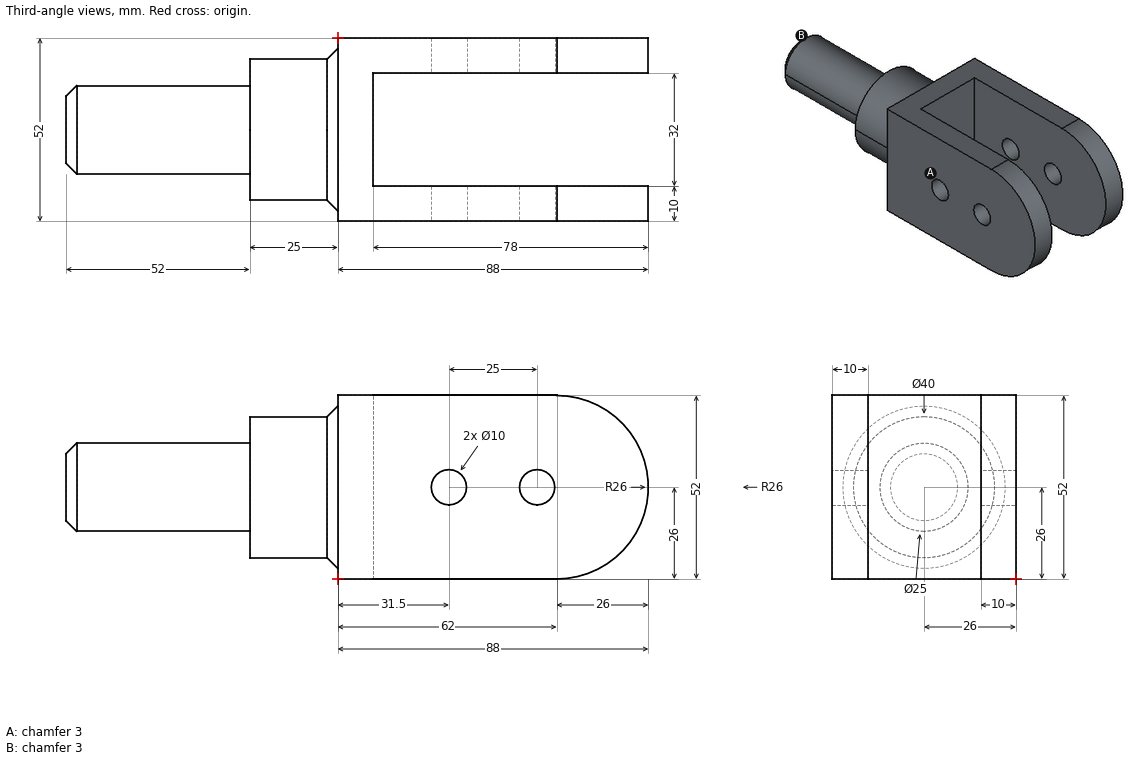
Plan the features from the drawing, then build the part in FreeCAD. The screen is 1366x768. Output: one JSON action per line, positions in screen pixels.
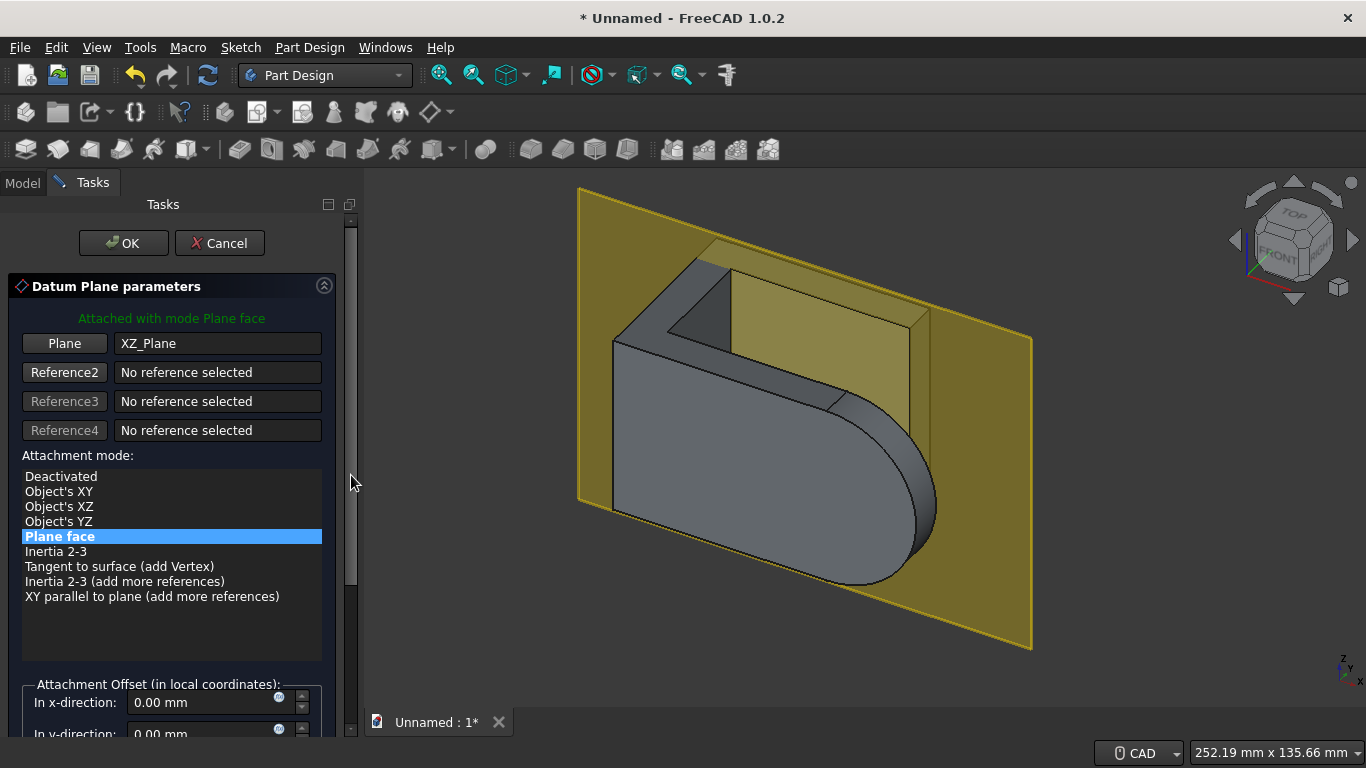
{"action": "left_click", "coordinate": [124, 243]}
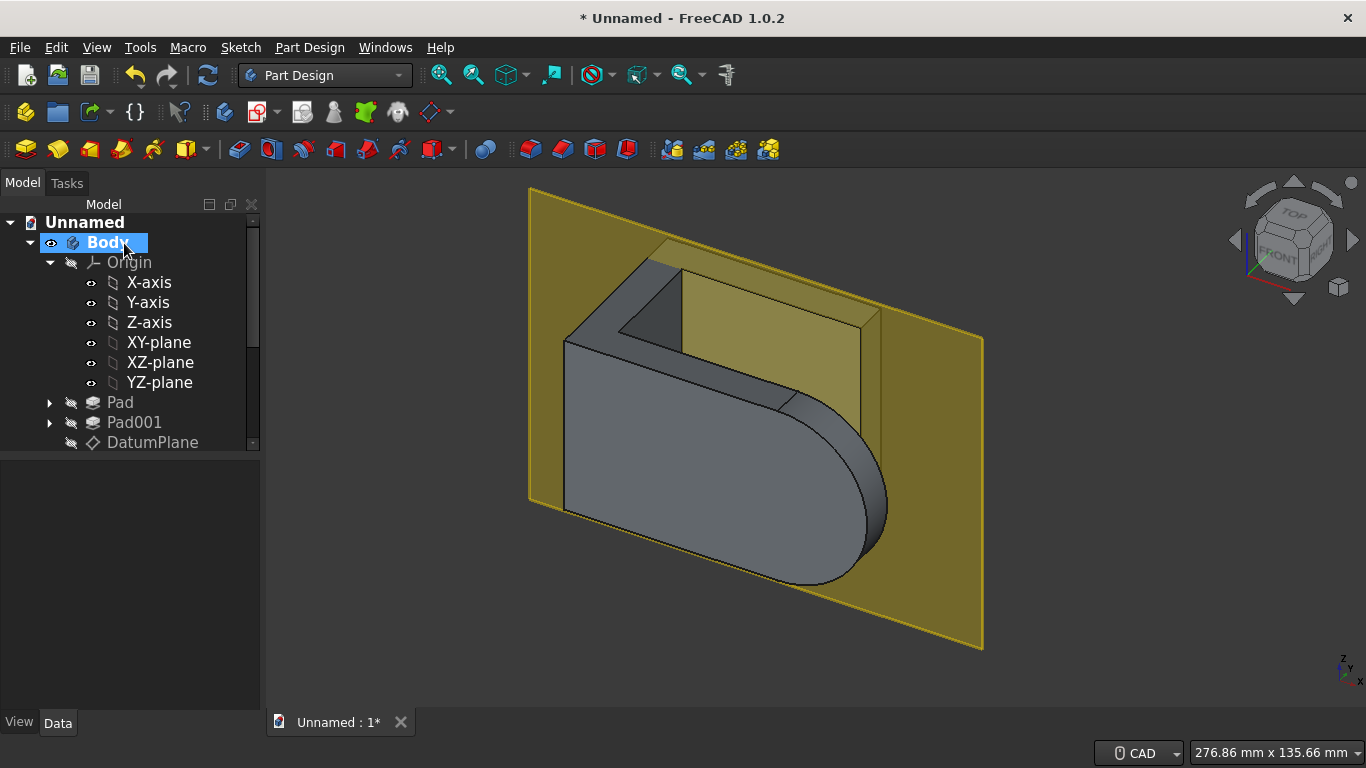
{"action": "scroll", "coordinate": [100, 338], "scroll_direction": "down", "scroll_amount": 3}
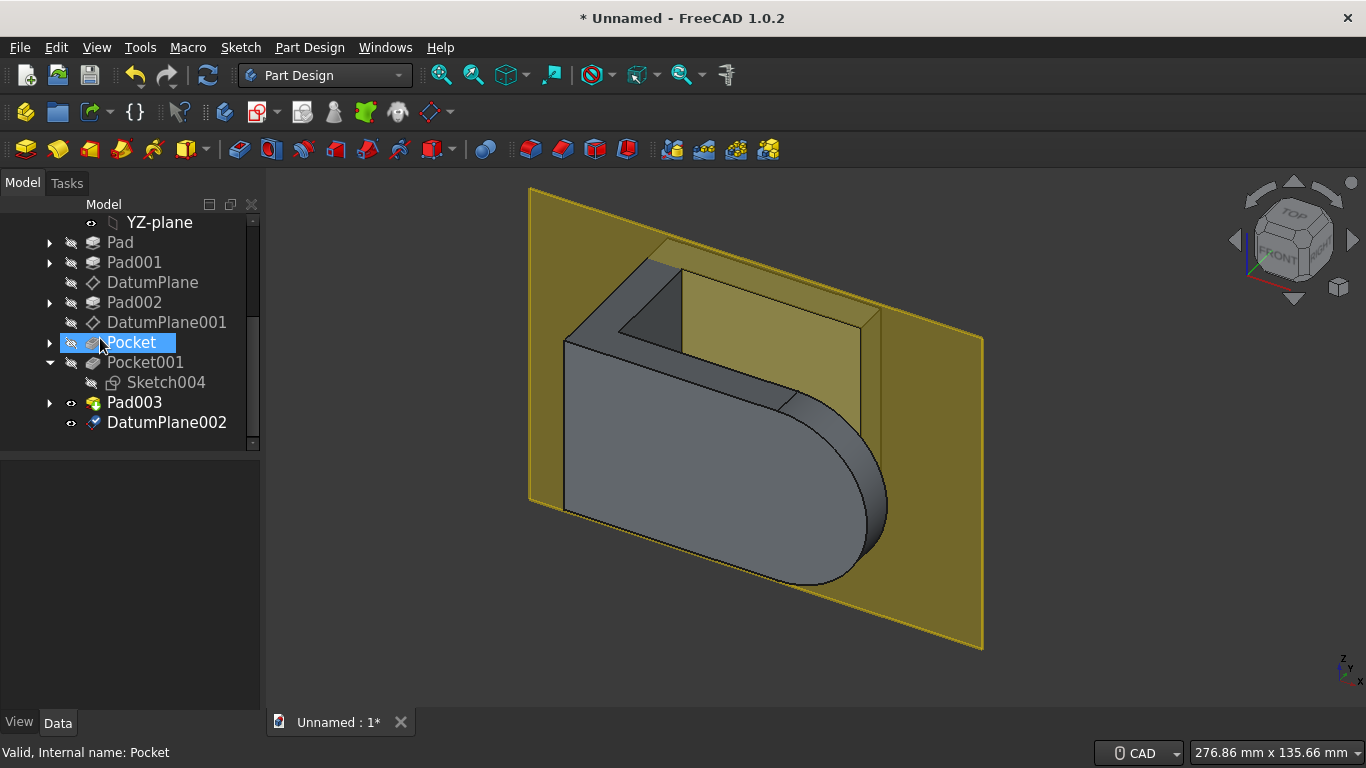
{"action": "left_click", "coordinate": [116, 423]}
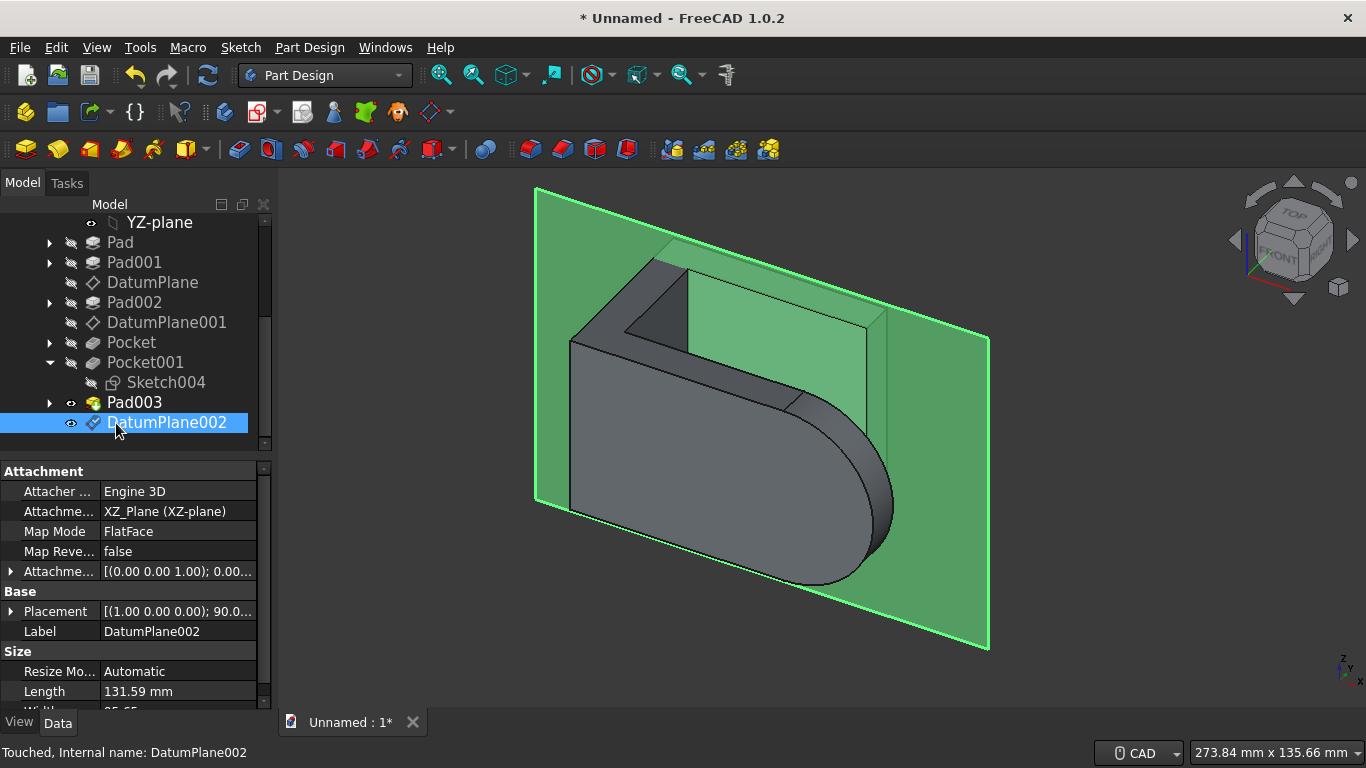
{"action": "left_click", "coordinate": [258, 112]}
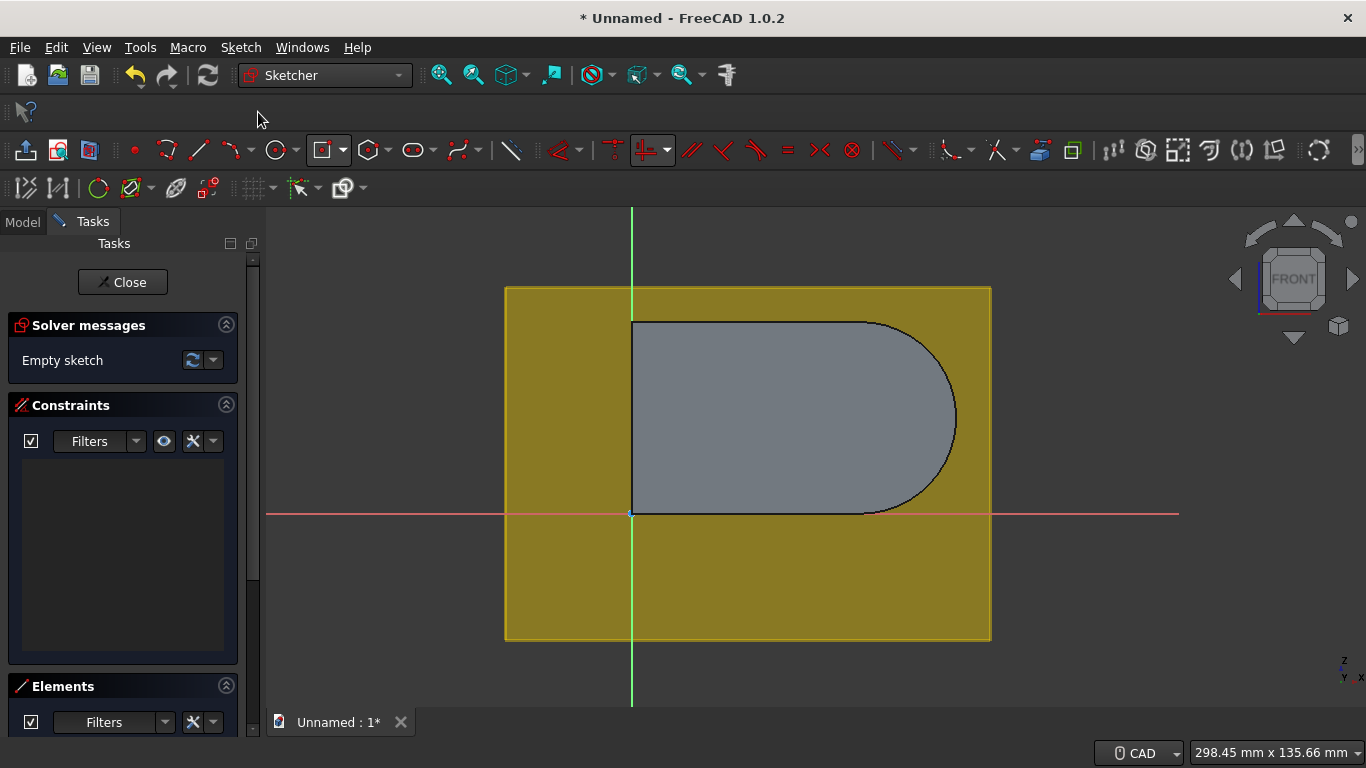
{"action": "left_click", "coordinate": [90, 150]}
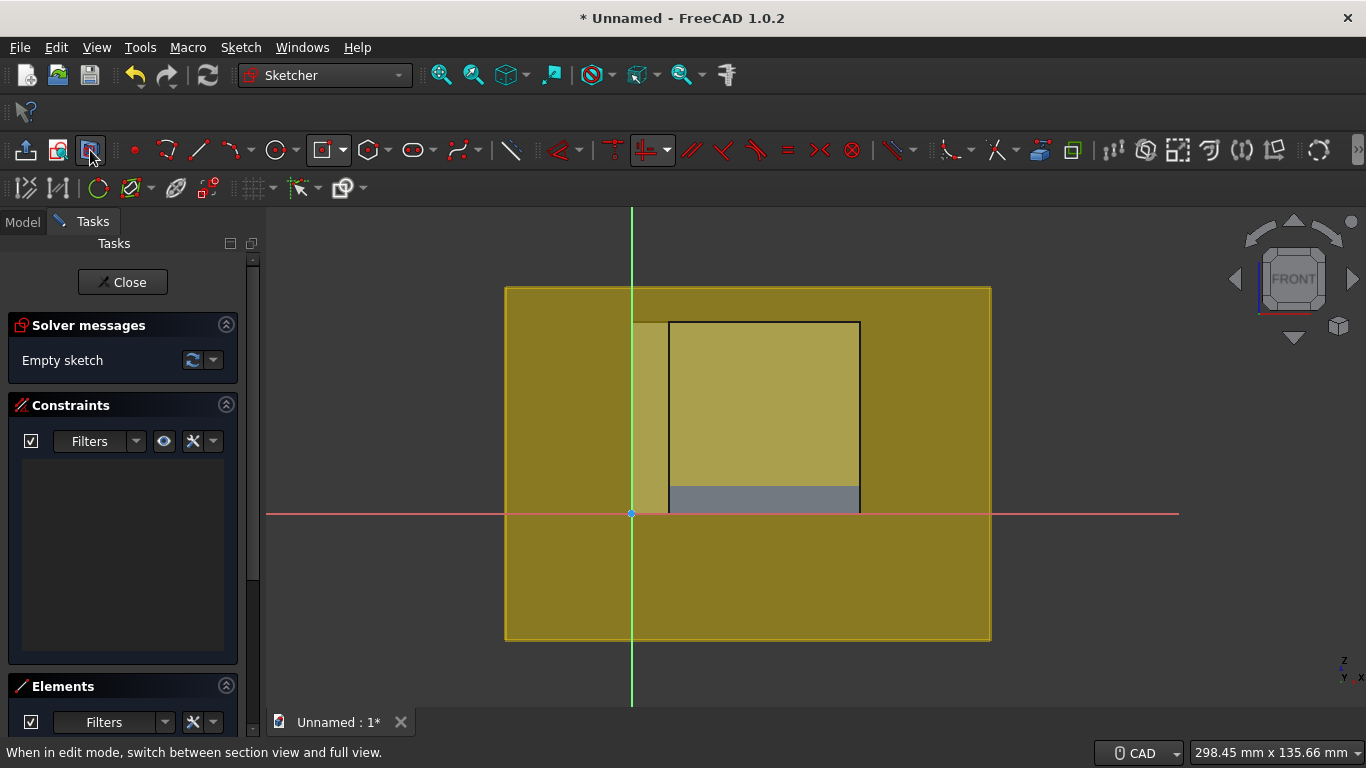
{"action": "scroll", "coordinate": [889, 338], "scroll_direction": "up", "scroll_amount": 2}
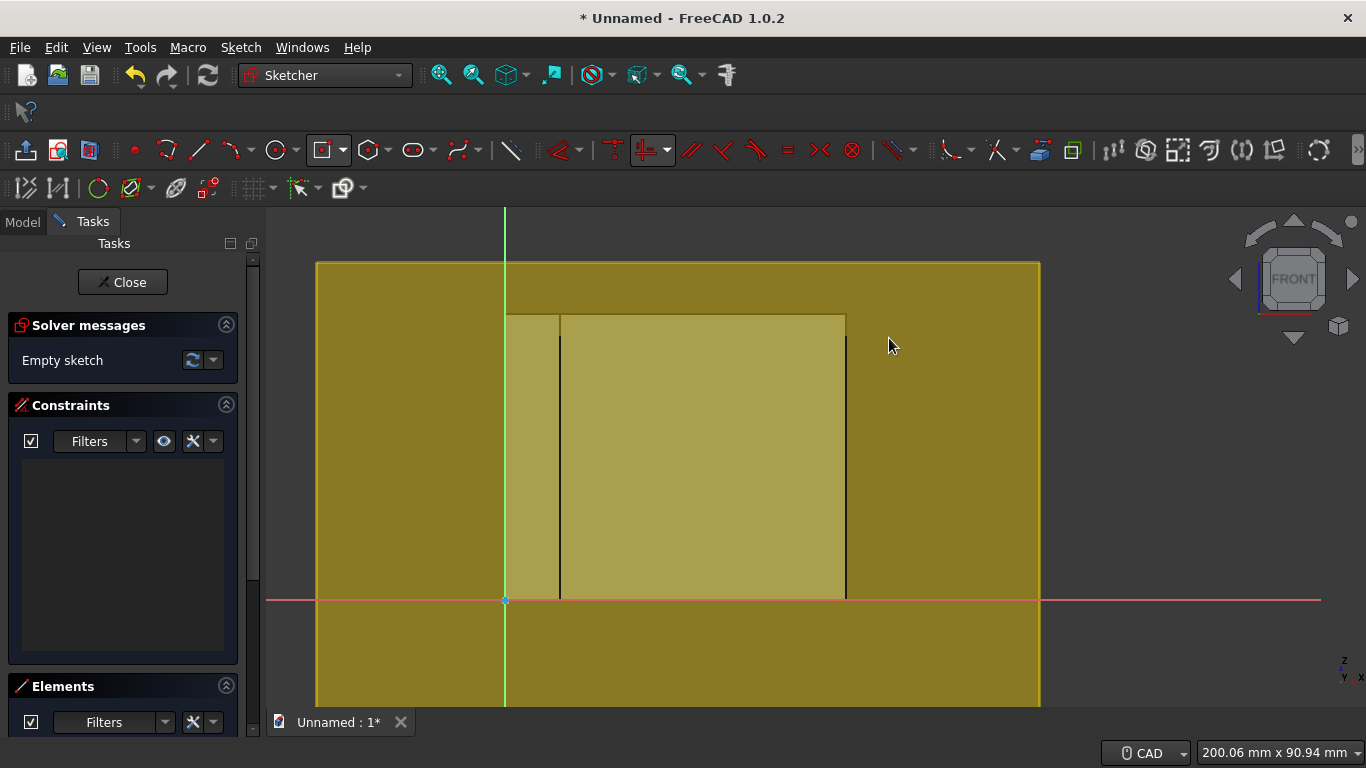
{"action": "left_click", "coordinate": [200, 150]}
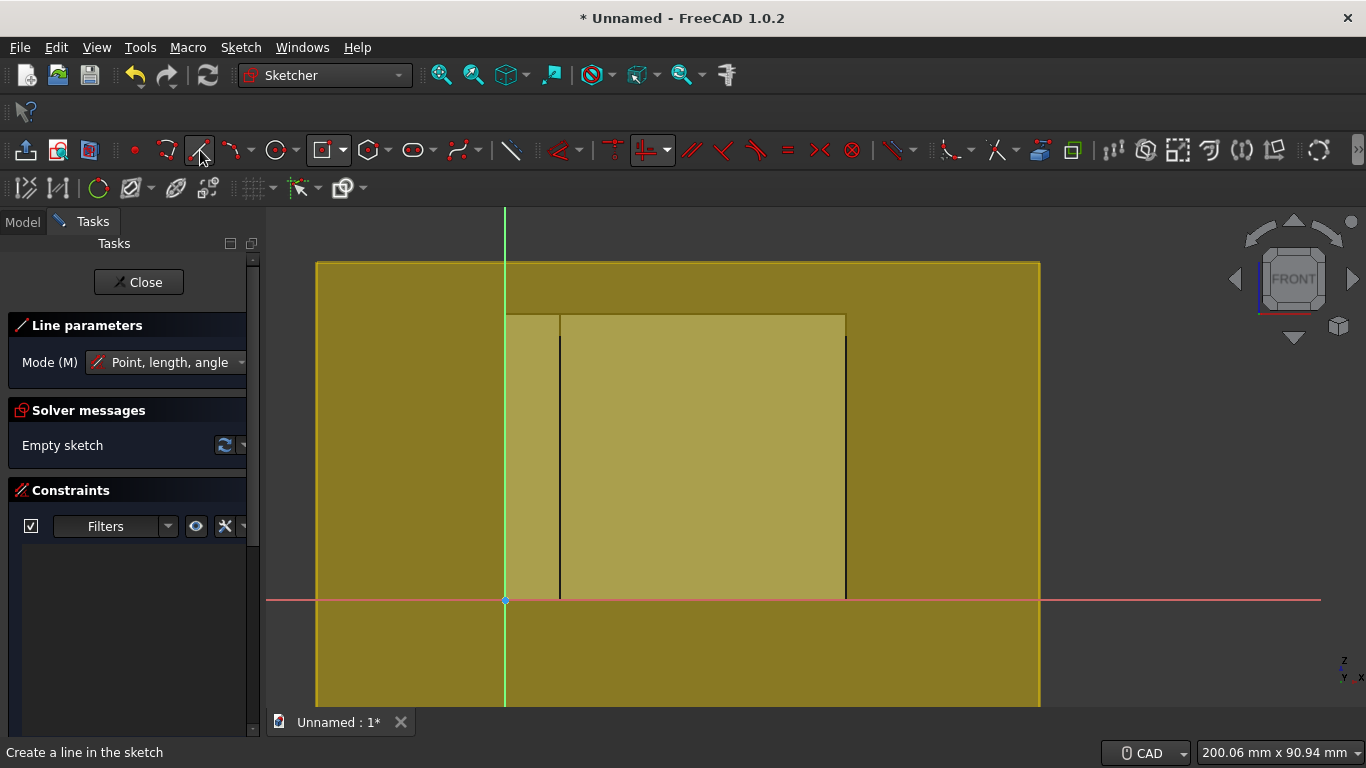
{"action": "left_click", "coordinate": [846, 600]}
{"action": "left_click", "coordinate": [846, 314]}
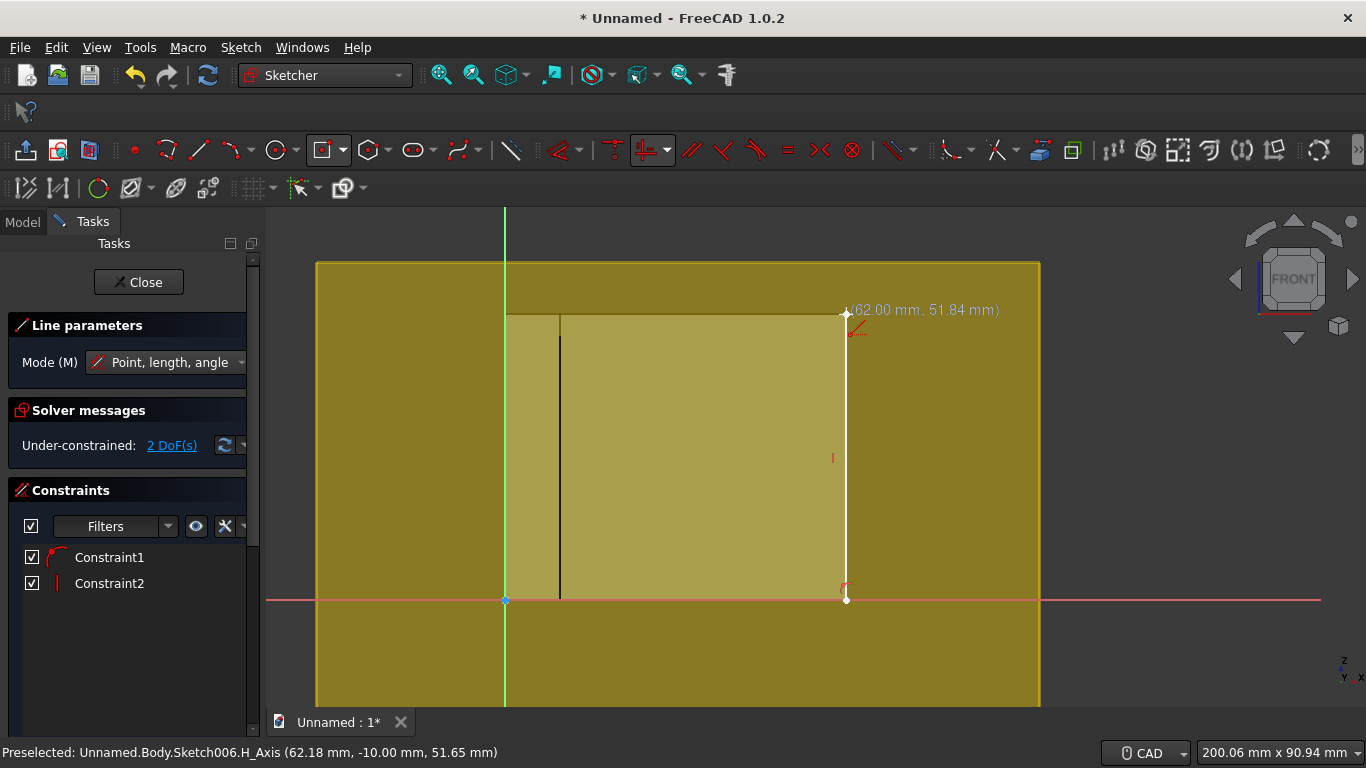
{"action": "left_click", "coordinate": [232, 150]}